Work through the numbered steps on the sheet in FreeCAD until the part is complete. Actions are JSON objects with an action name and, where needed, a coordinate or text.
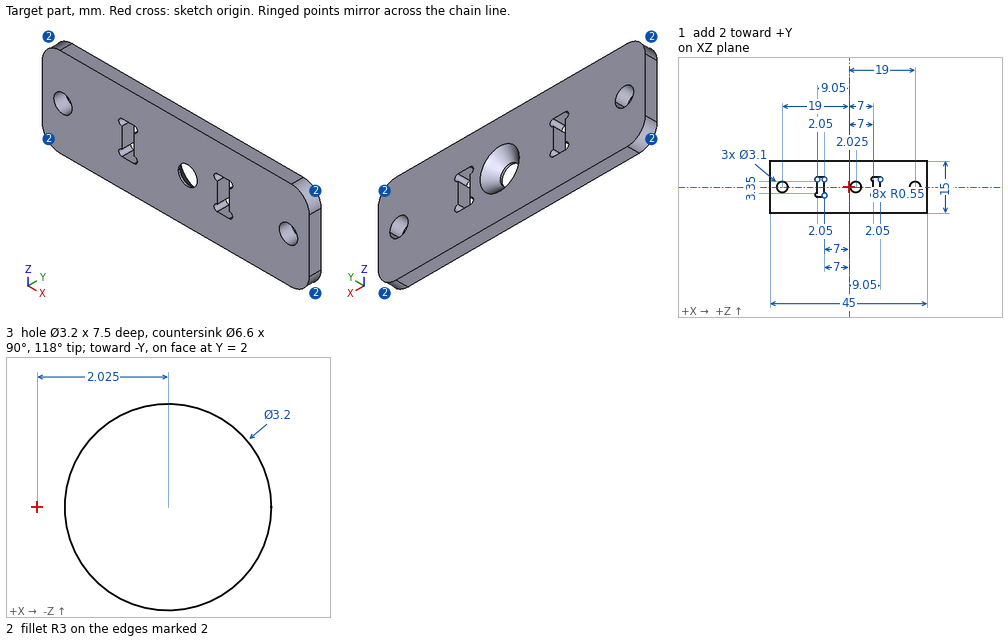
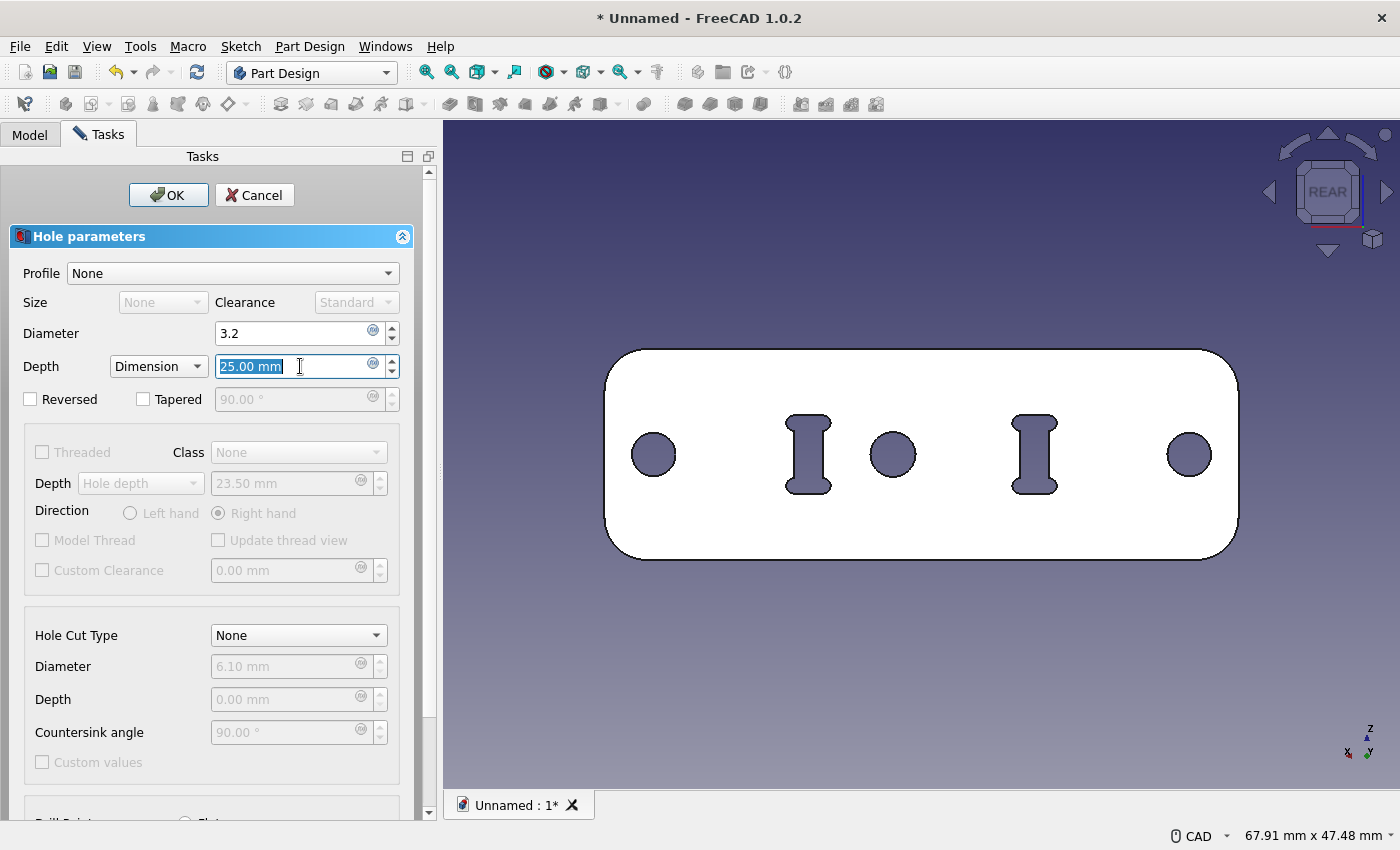
{"action": "type", "text": "7.5"}
{"action": "key", "text": "Tab"}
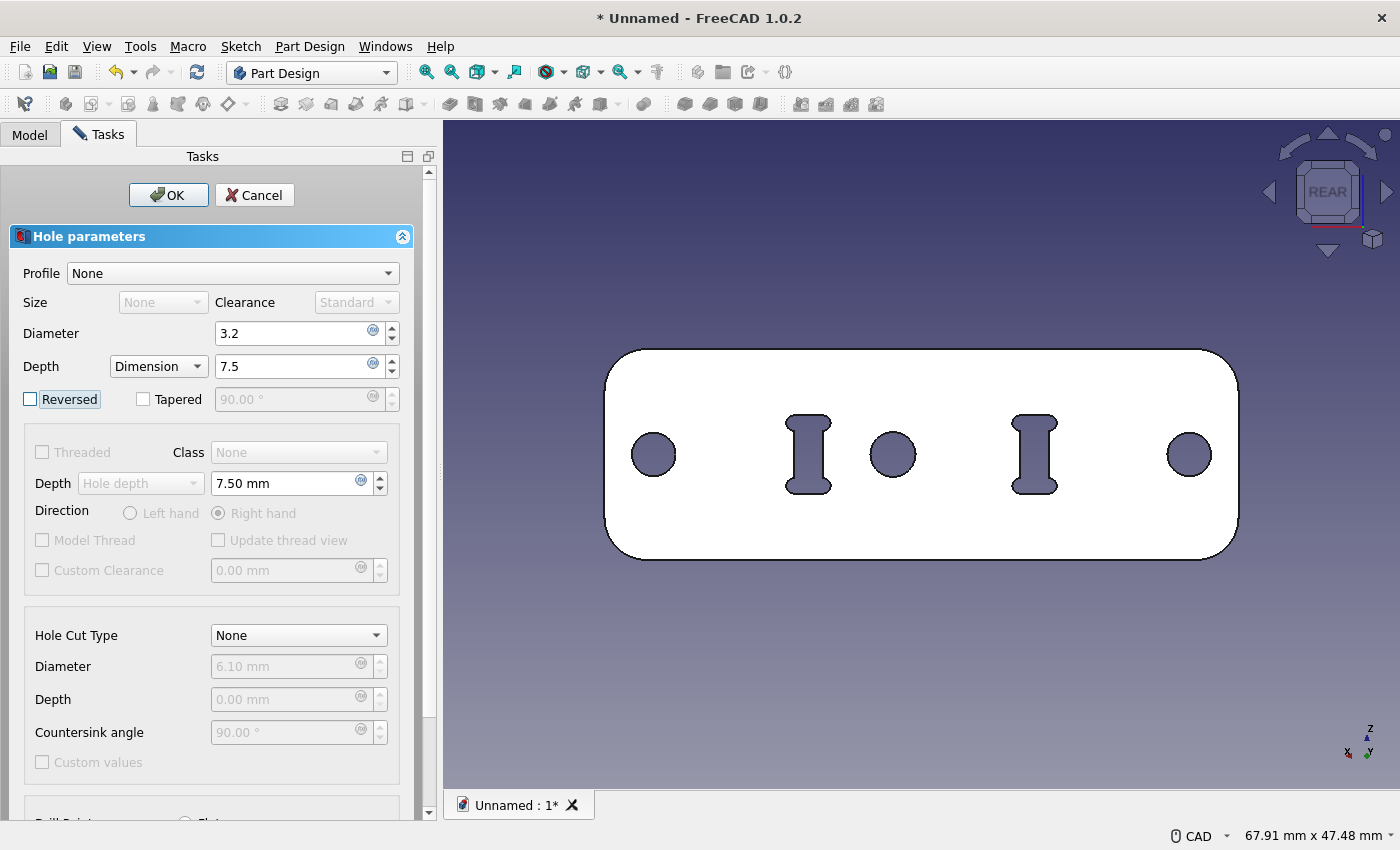
{"action": "left_click", "coordinate": [300, 636]}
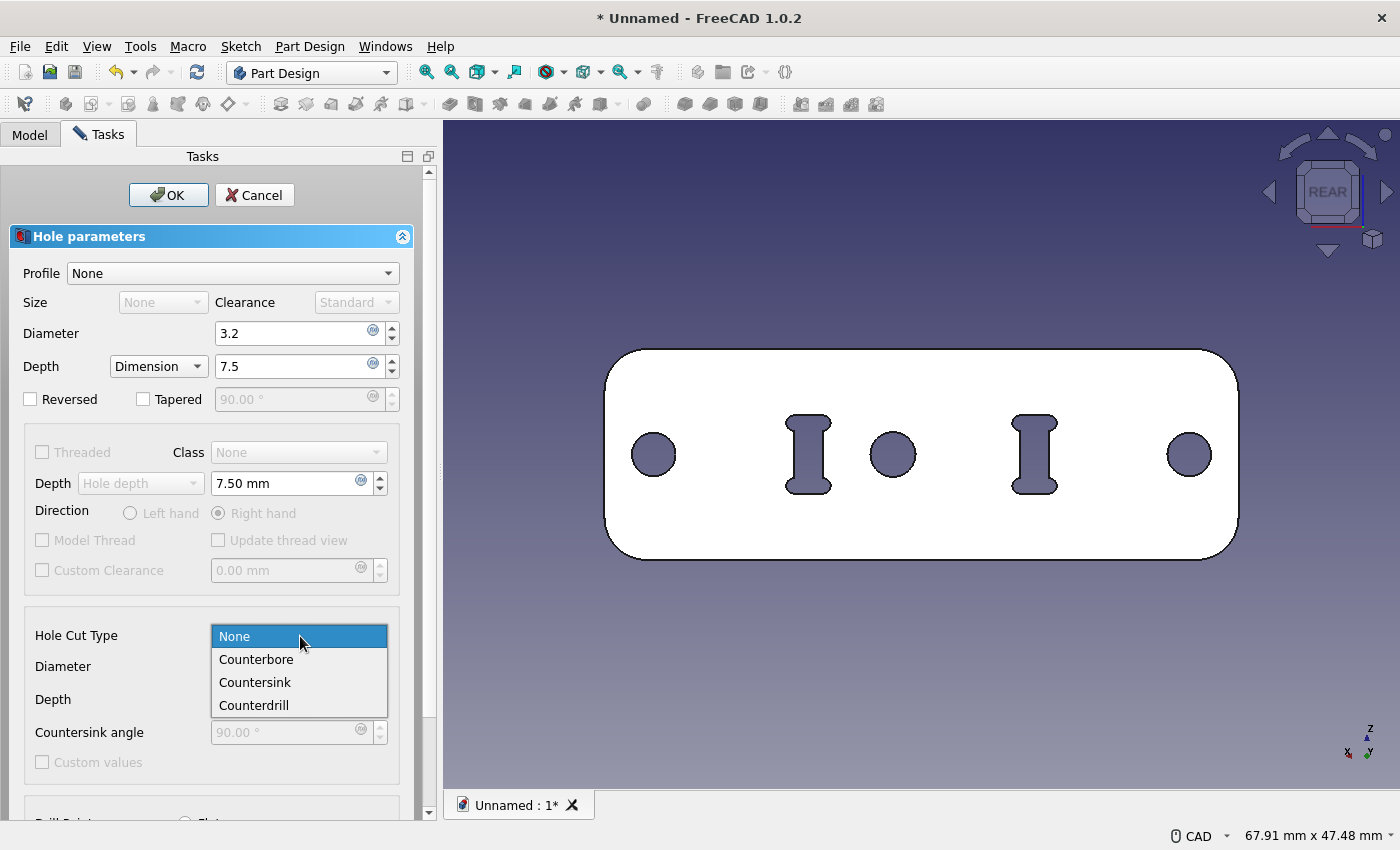
{"action": "left_click", "coordinate": [298, 682]}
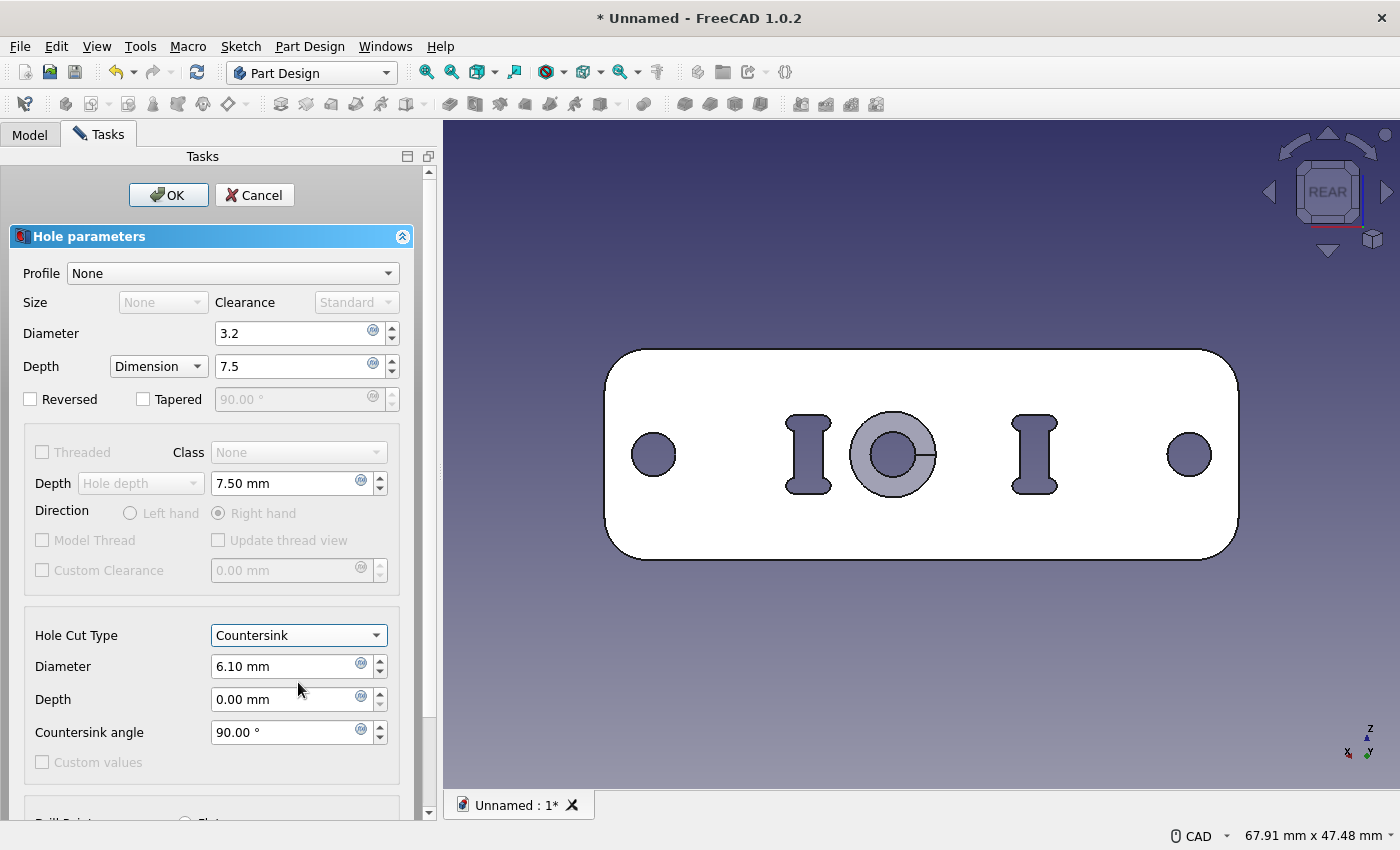
{"action": "triple_click", "coordinate": [292, 666]}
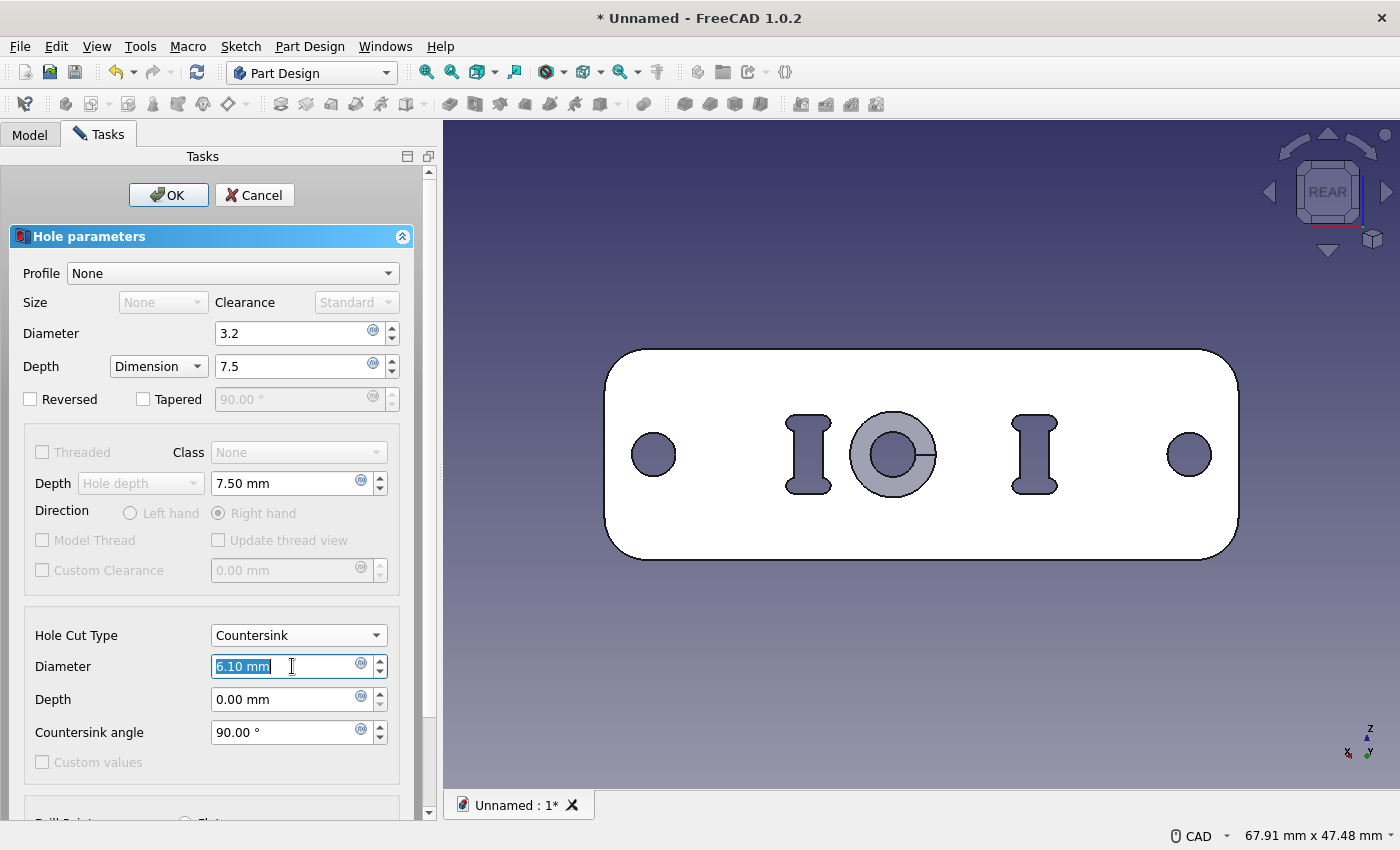
{"action": "type", "text": "6.6"}
{"action": "key", "text": "Tab"}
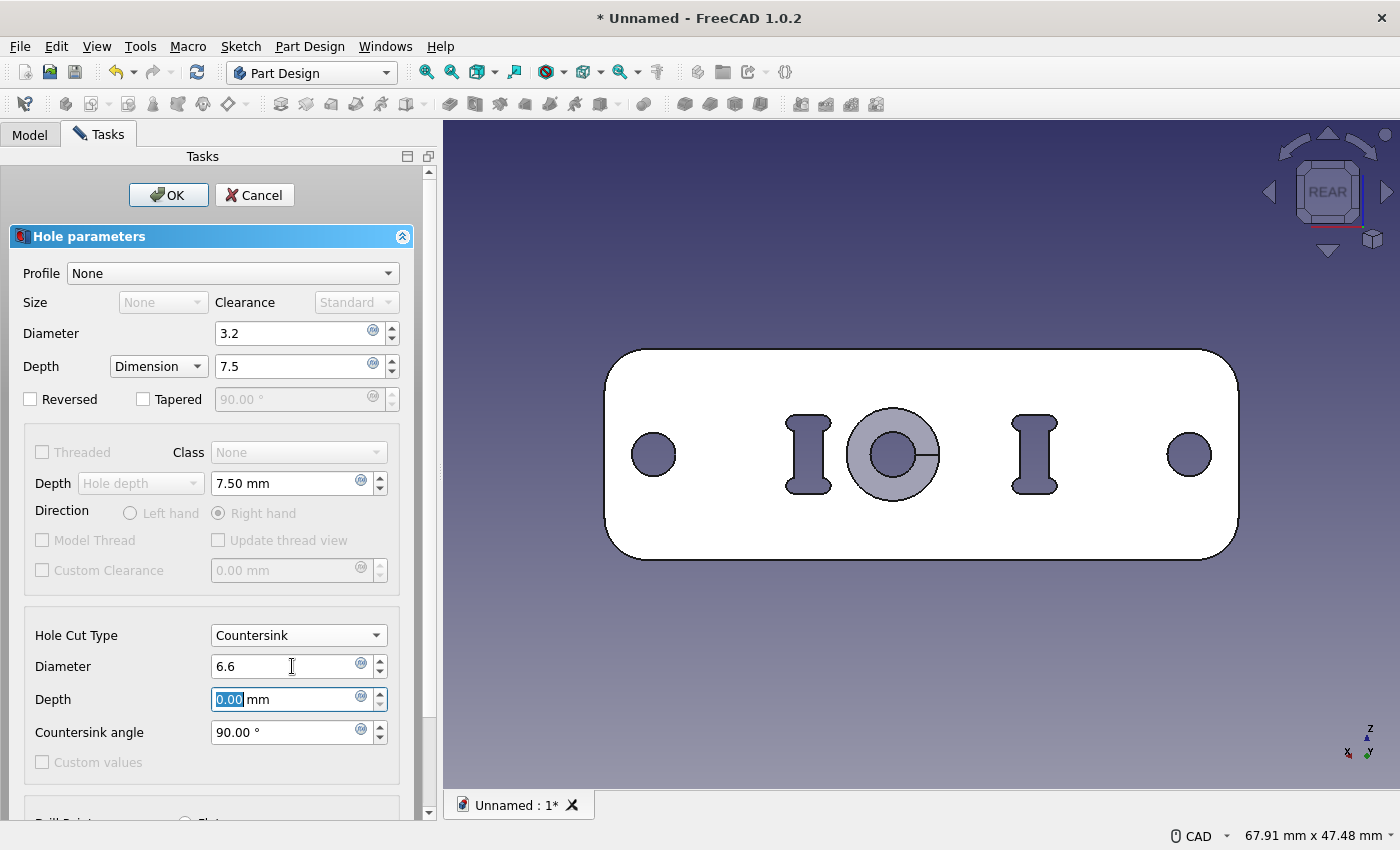
{"action": "left_click", "coordinate": [169, 195]}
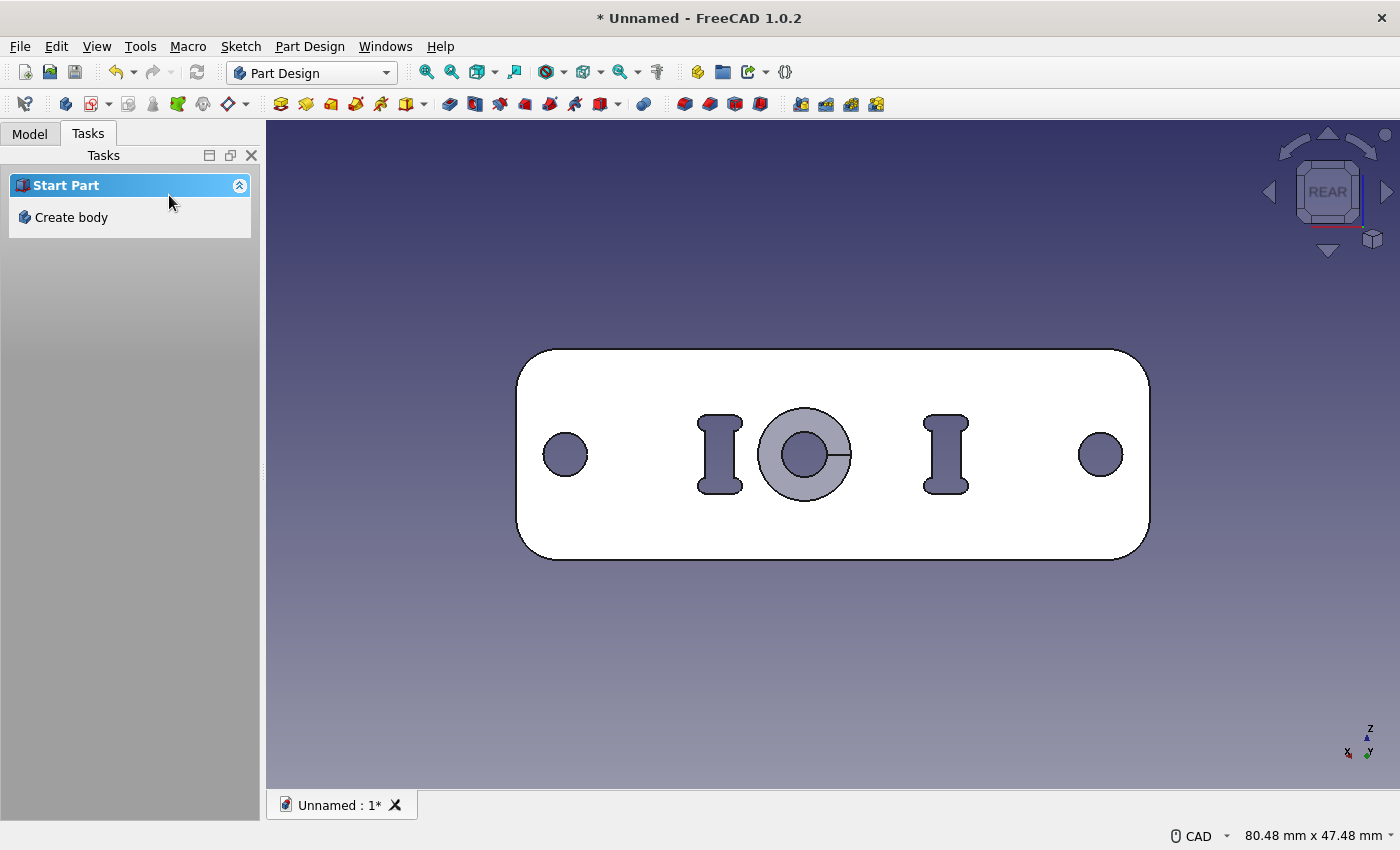
{"action": "key", "text": "0"}